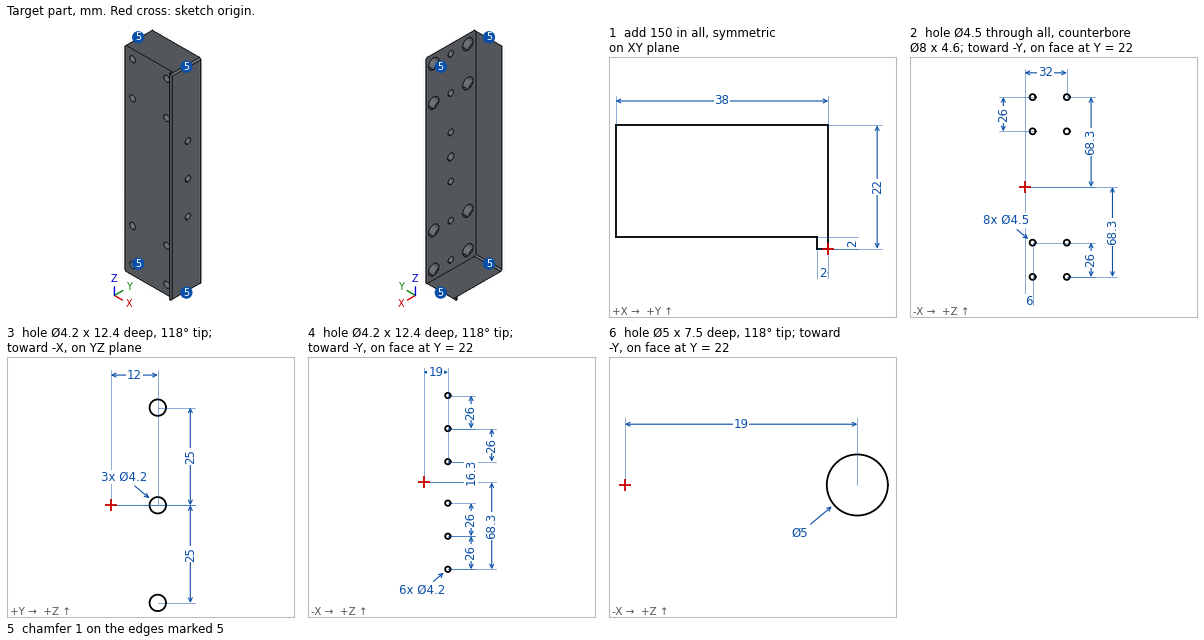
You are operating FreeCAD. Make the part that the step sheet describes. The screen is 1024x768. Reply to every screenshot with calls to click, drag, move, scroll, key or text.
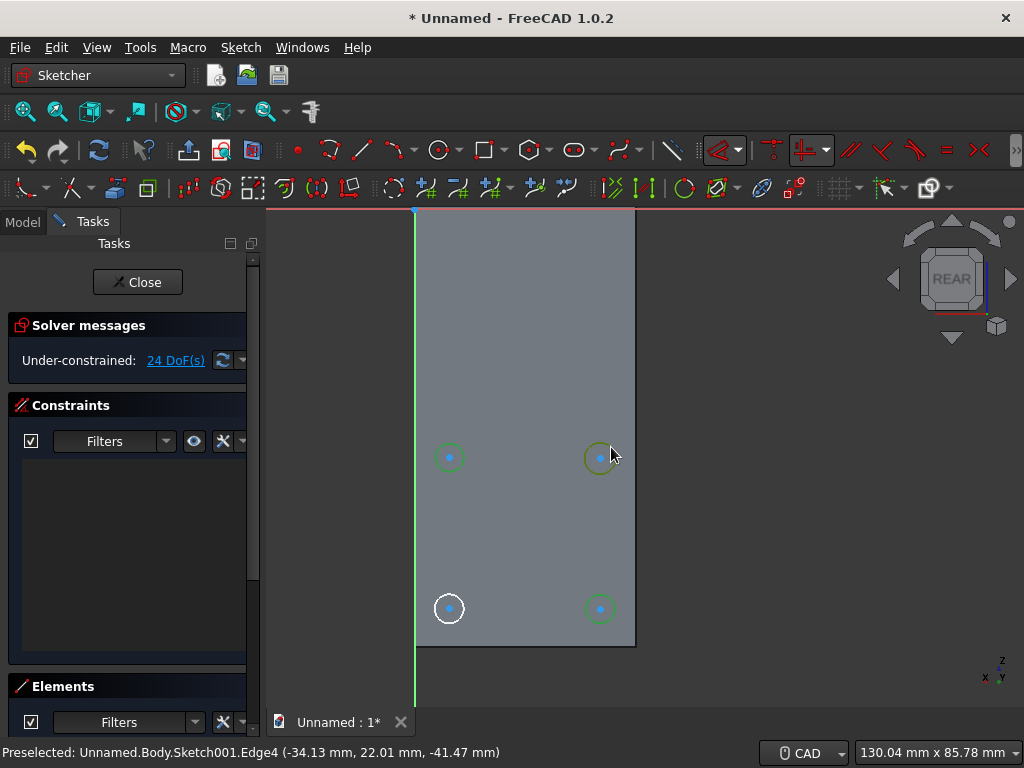
click(459, 599)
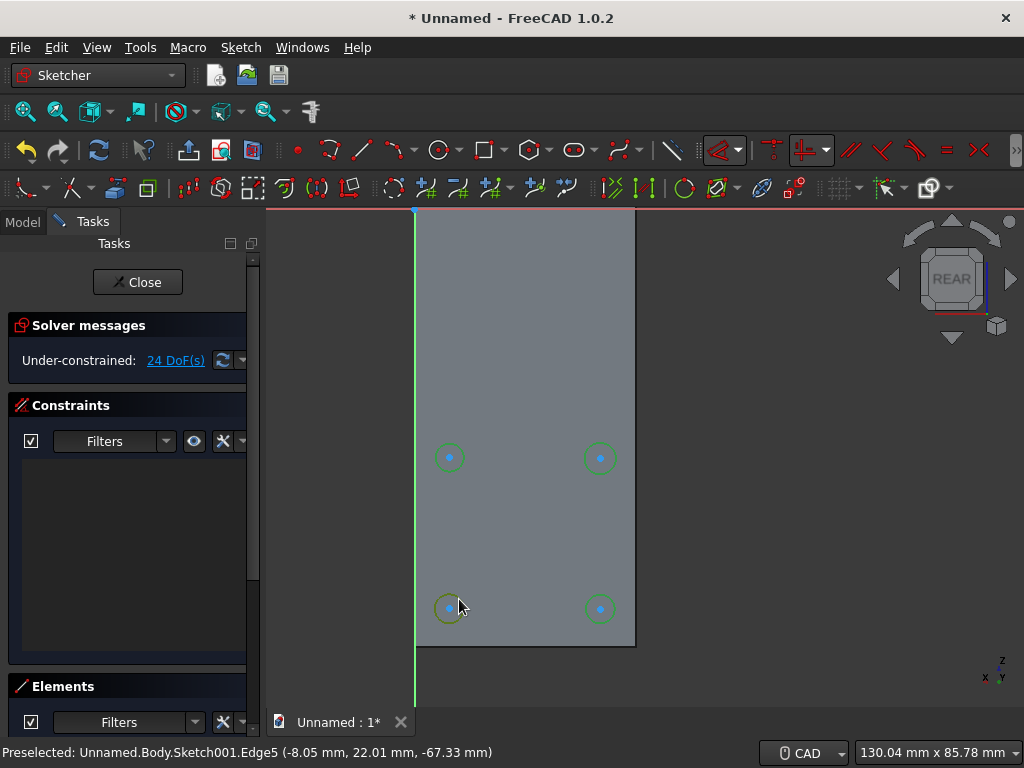
scroll(612, 601, down, 5)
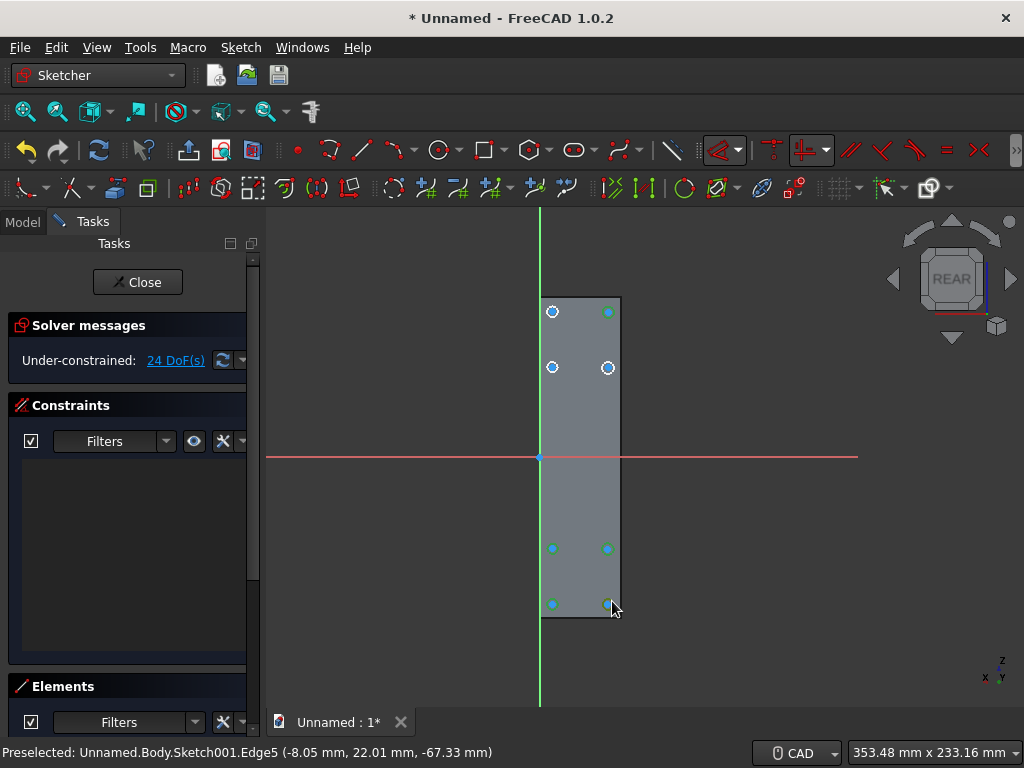
scroll(556, 308, up, 5)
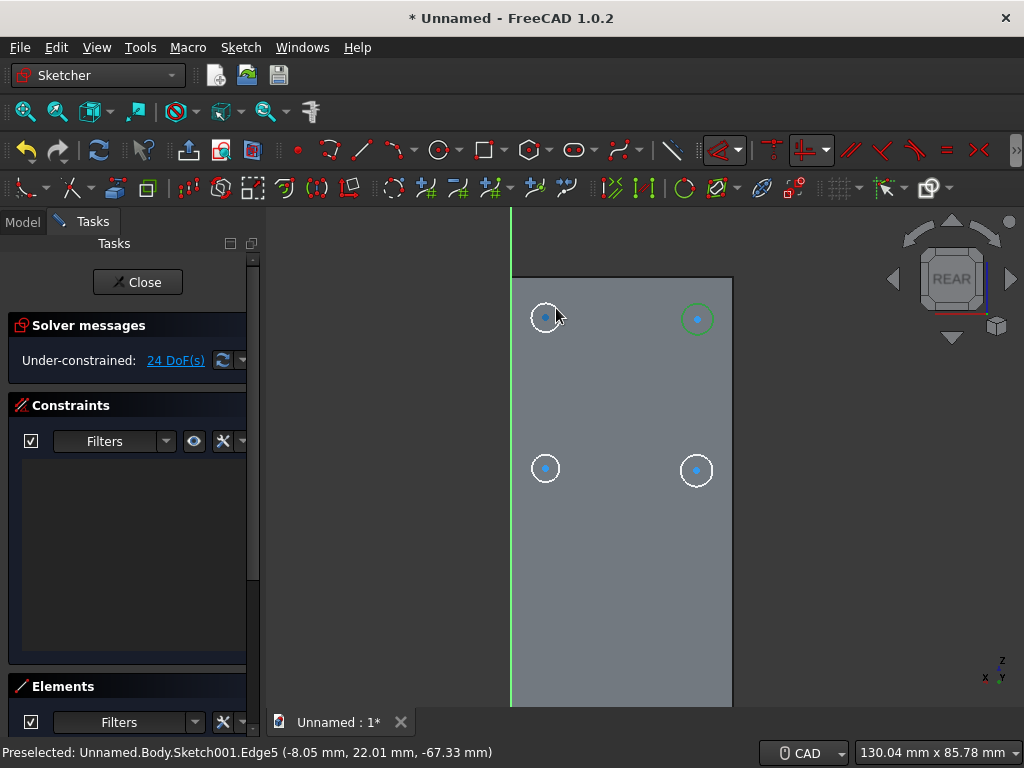
click(556, 308)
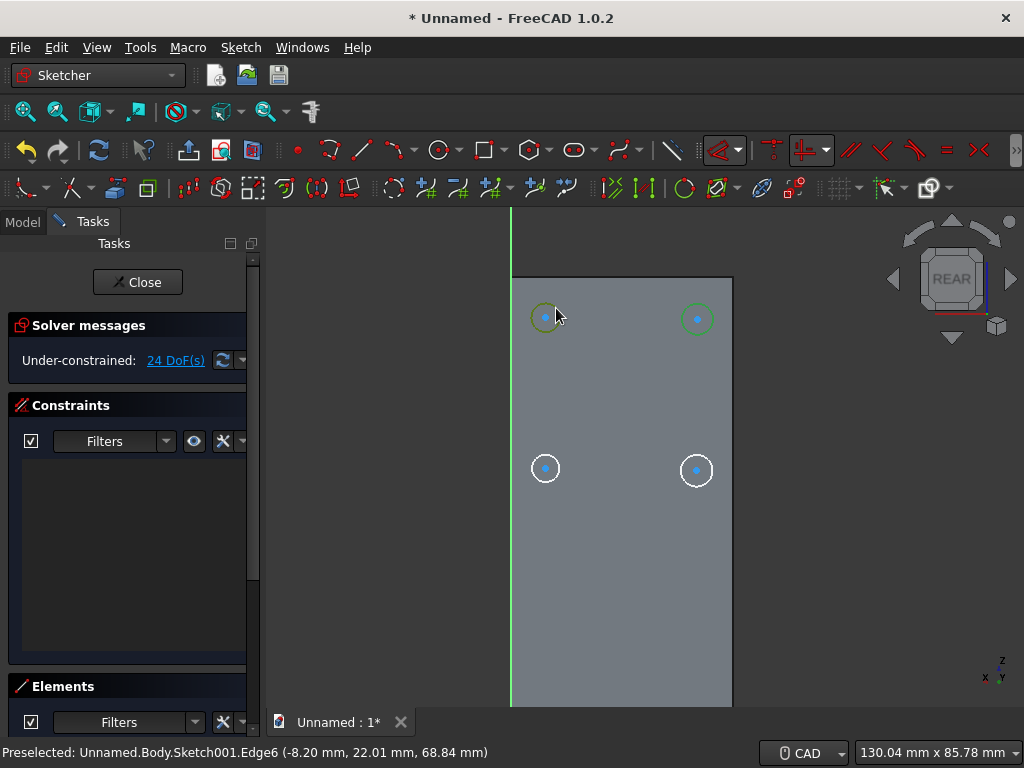
click(555, 459)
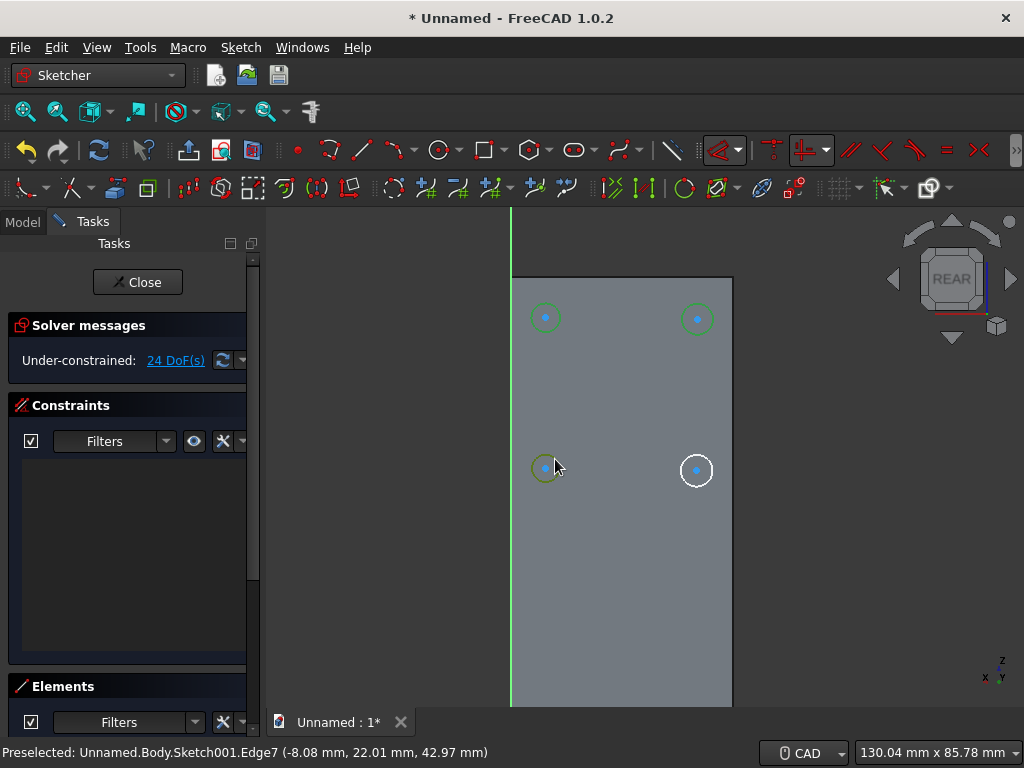
click(708, 460)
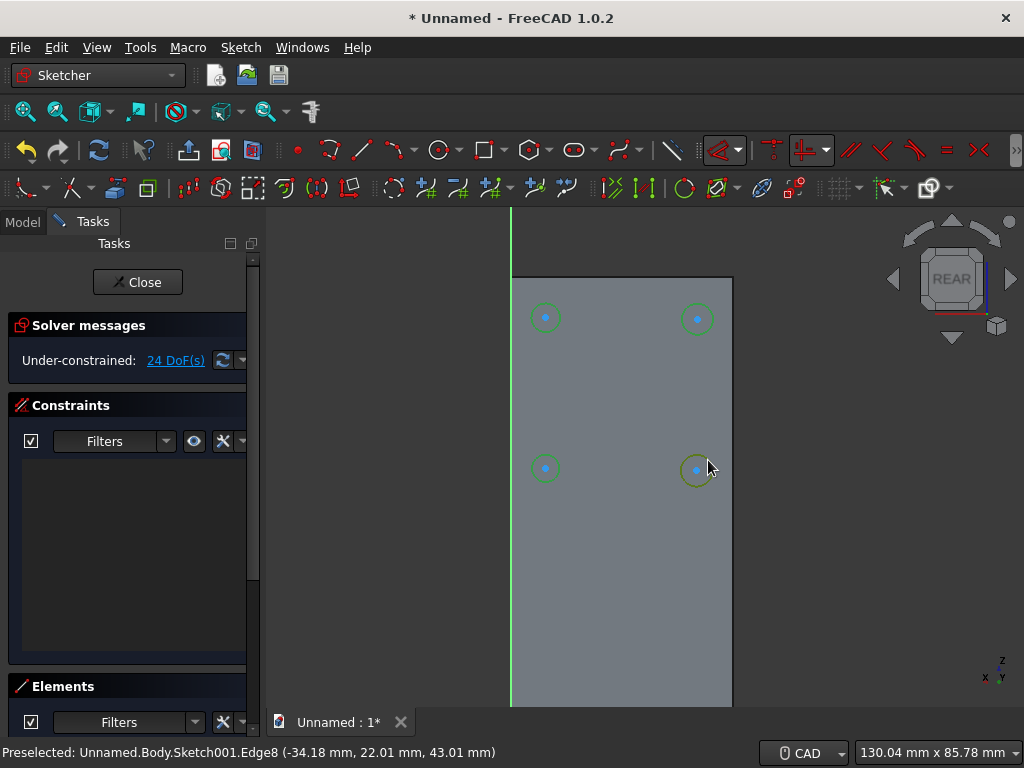
key(e)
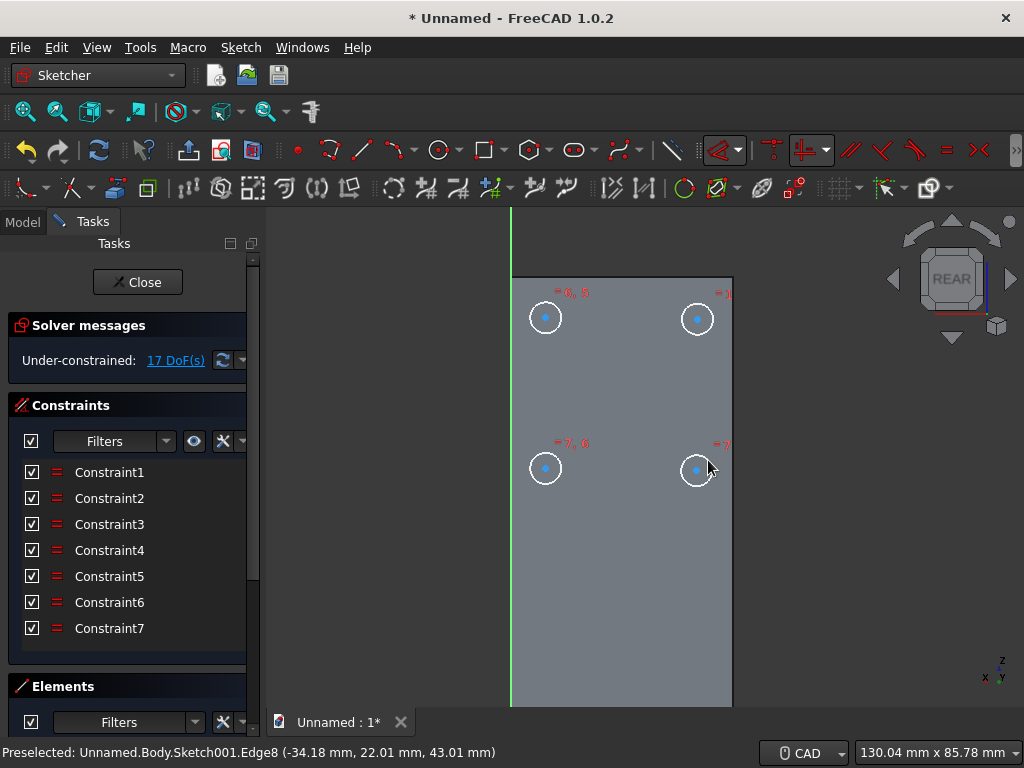
click(697, 319)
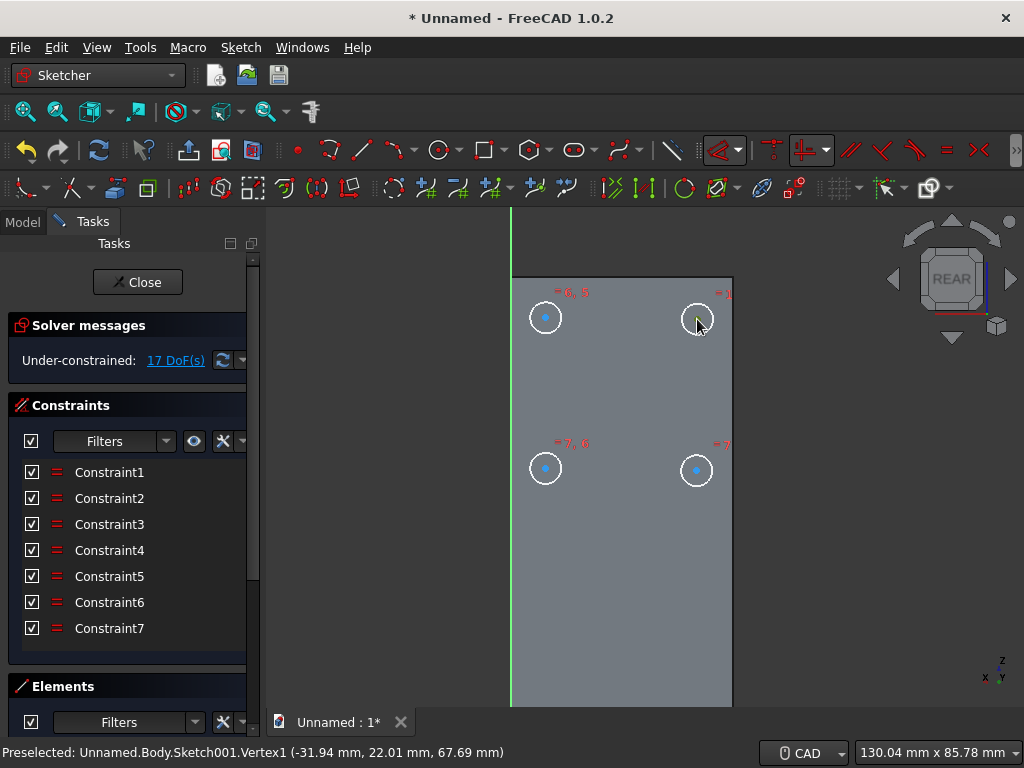
scroll(556, 308, down, 5)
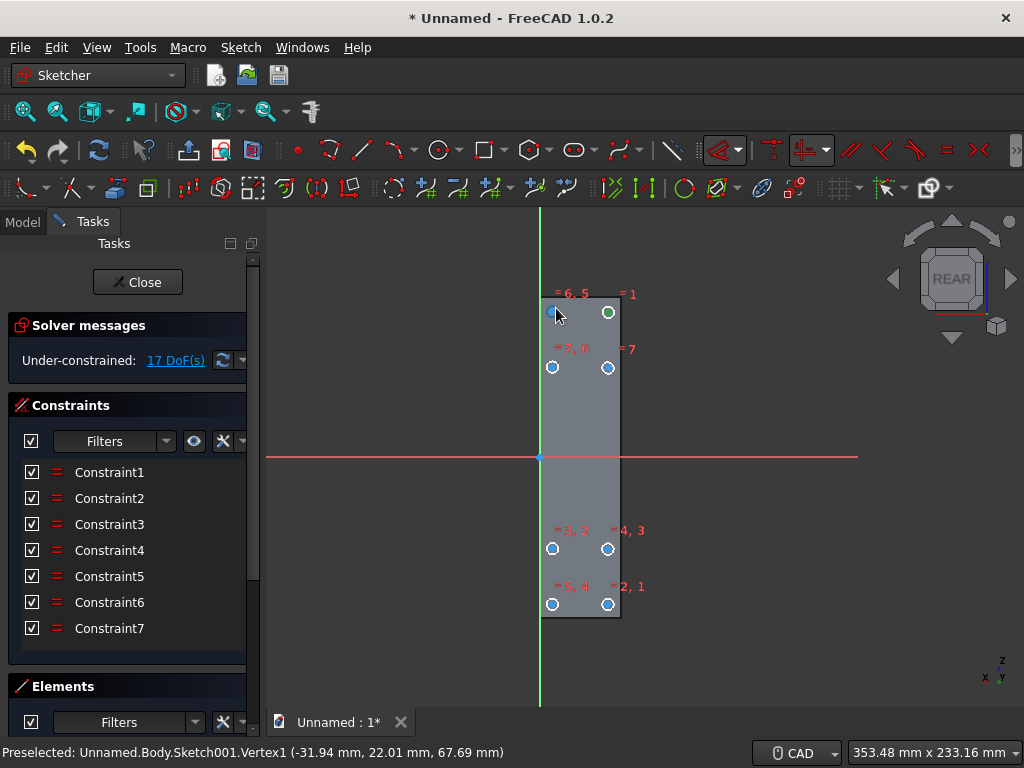
click(608, 604)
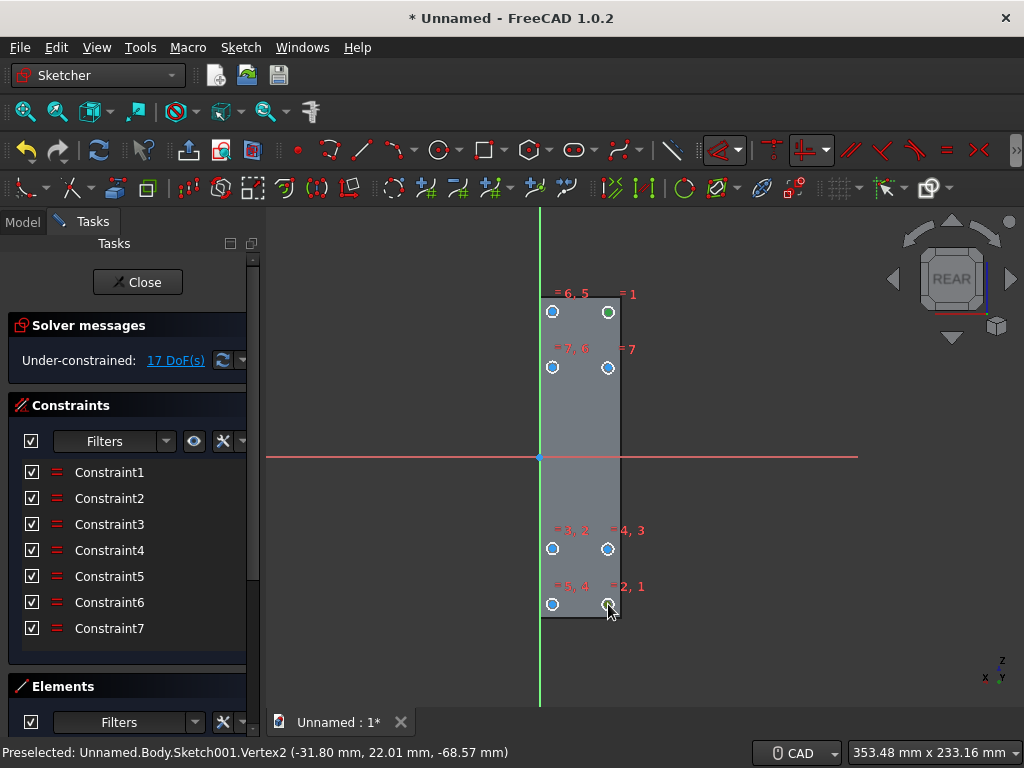
key(v)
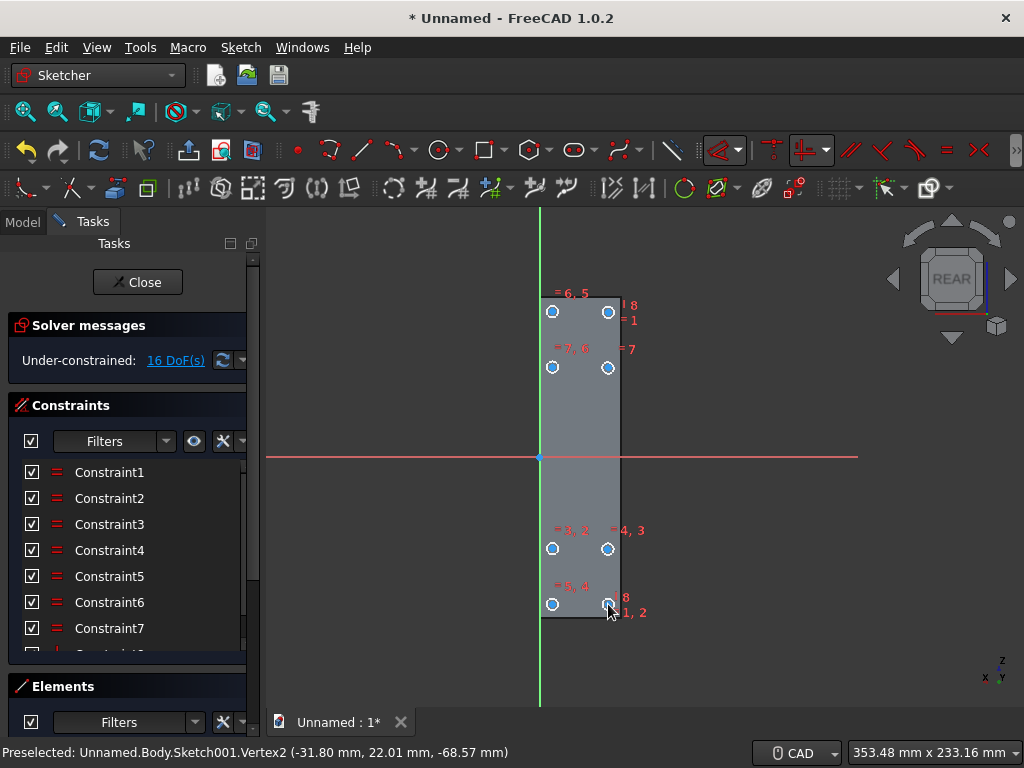
click(608, 604)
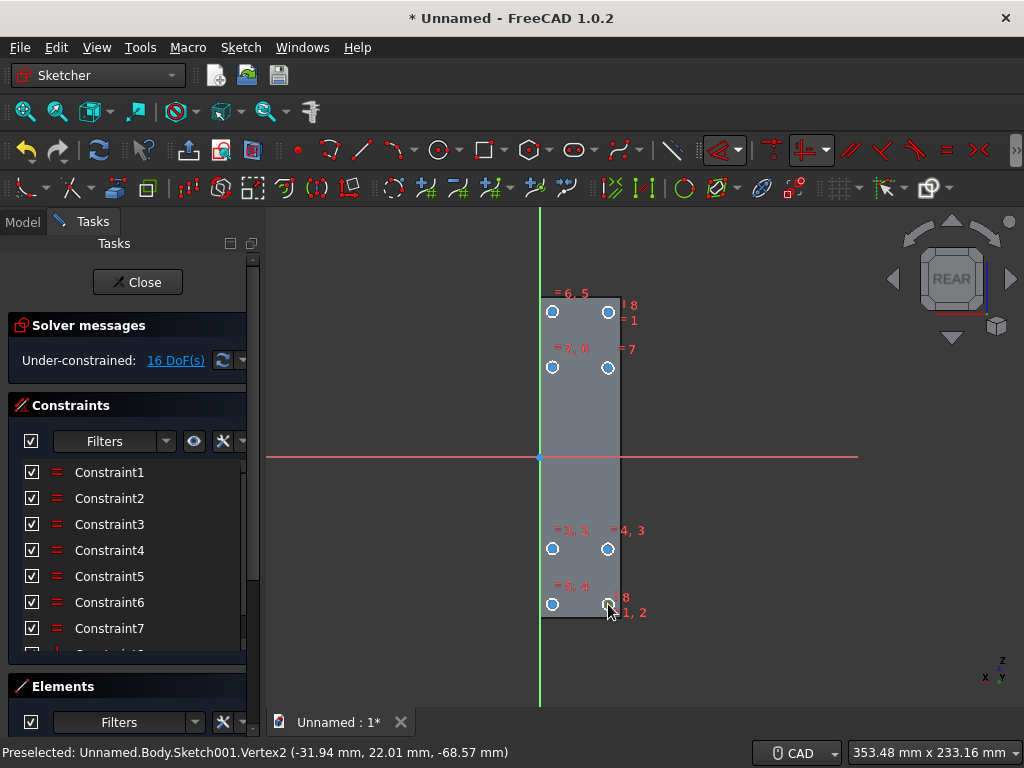
click(608, 549)